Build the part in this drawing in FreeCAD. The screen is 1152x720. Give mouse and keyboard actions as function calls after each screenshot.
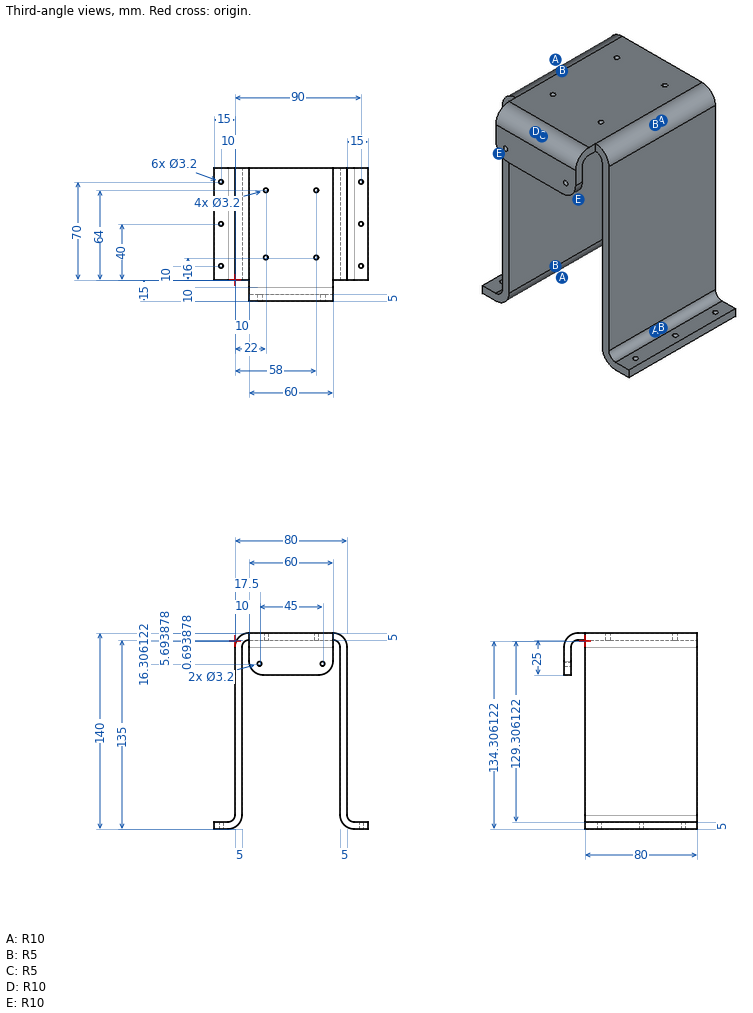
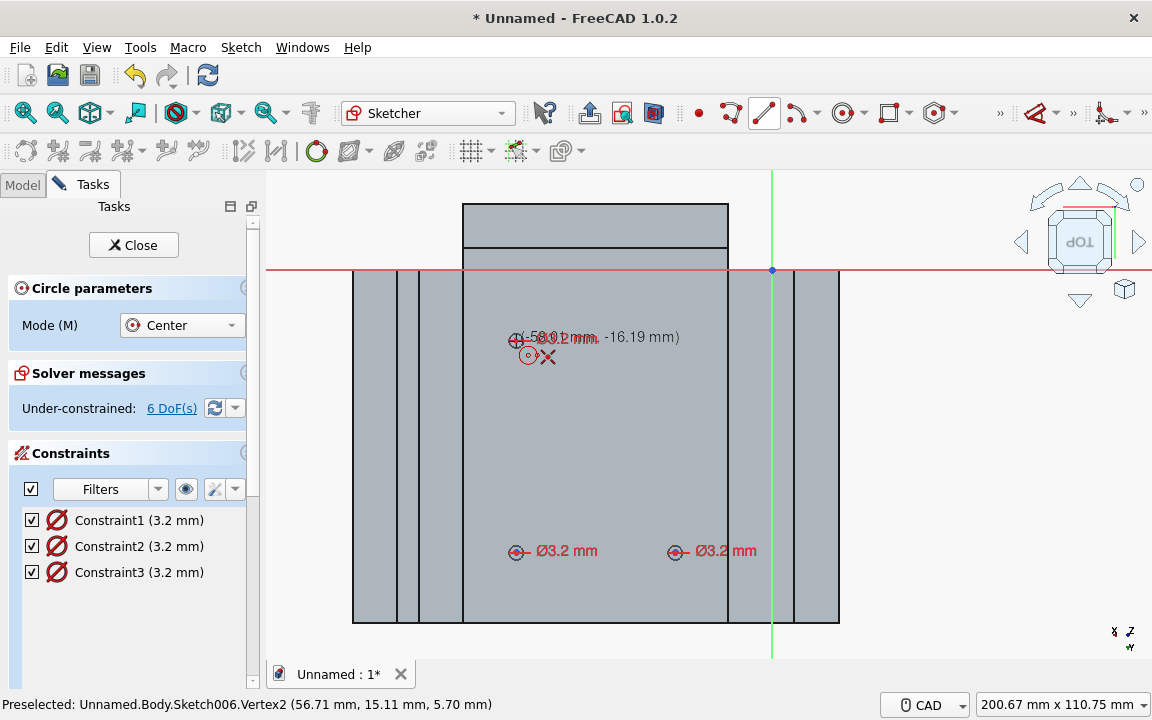
scroll(675, 341, up, 6)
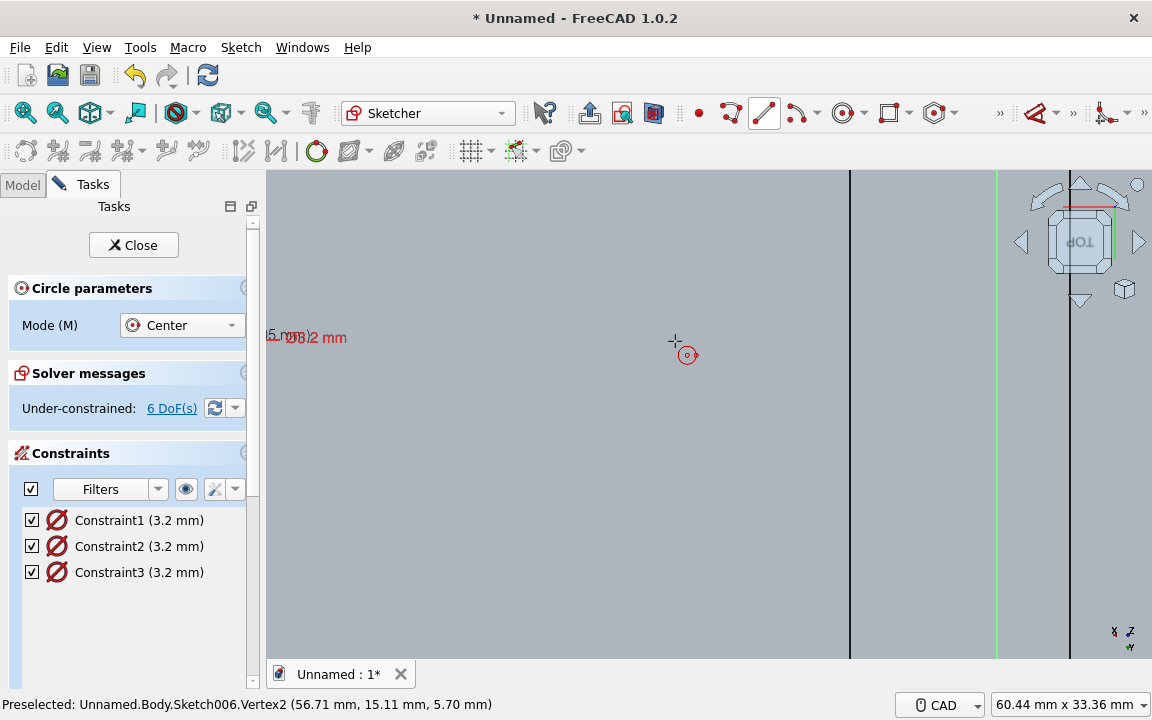
click(675, 339)
move(691, 323)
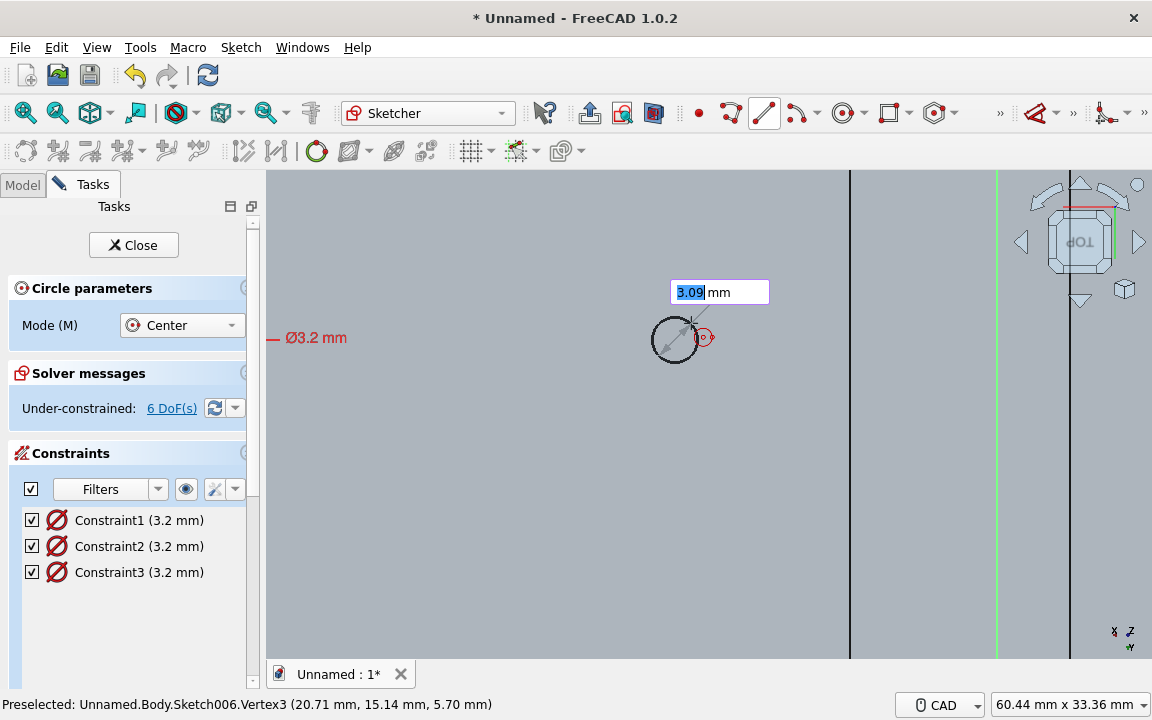
text(3.2)
key(Return)
key(Escape)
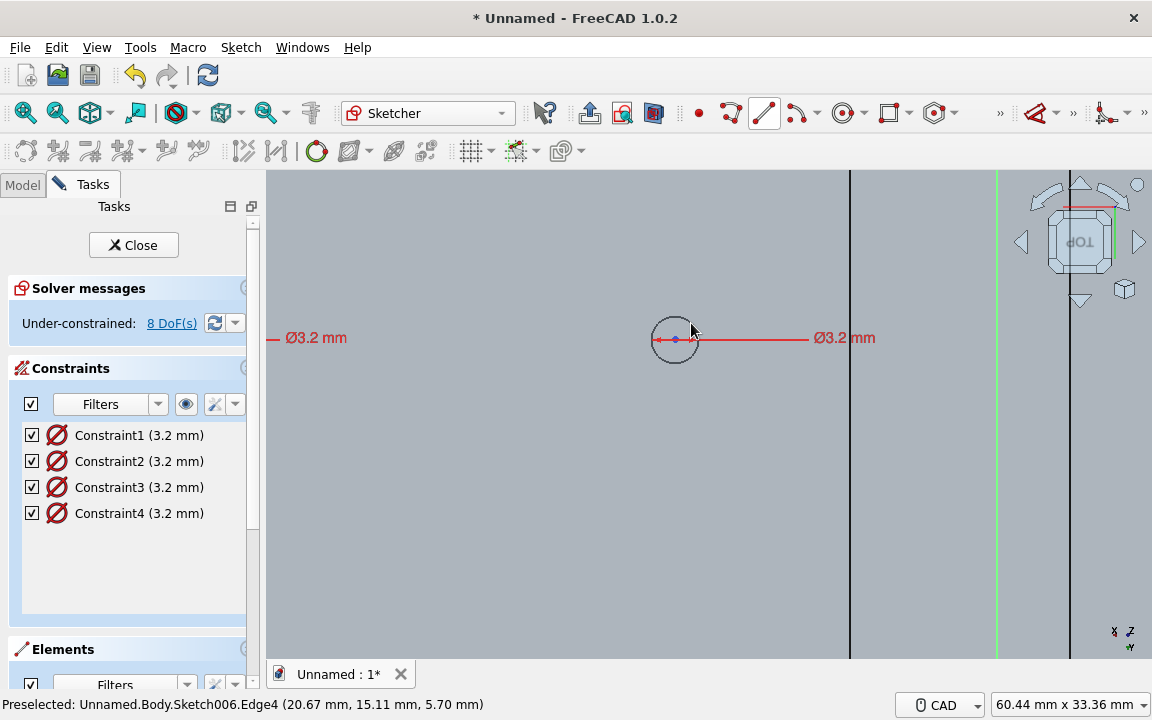
click(1036, 114)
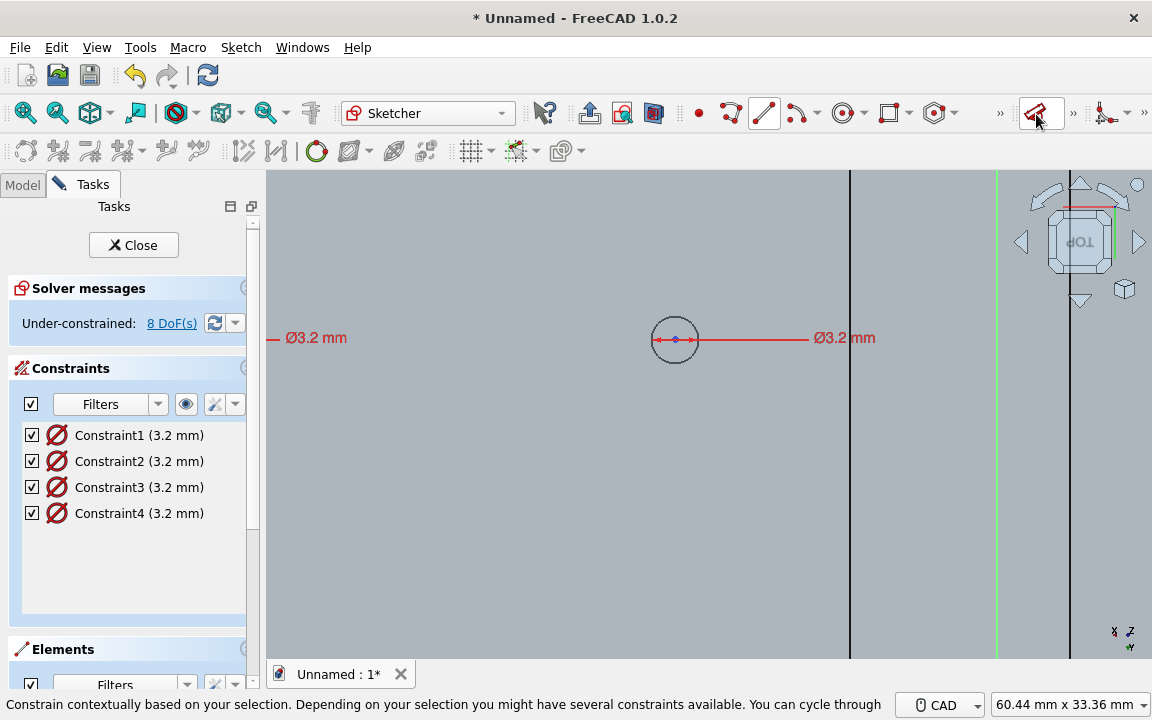
scroll(675, 341, down, 6)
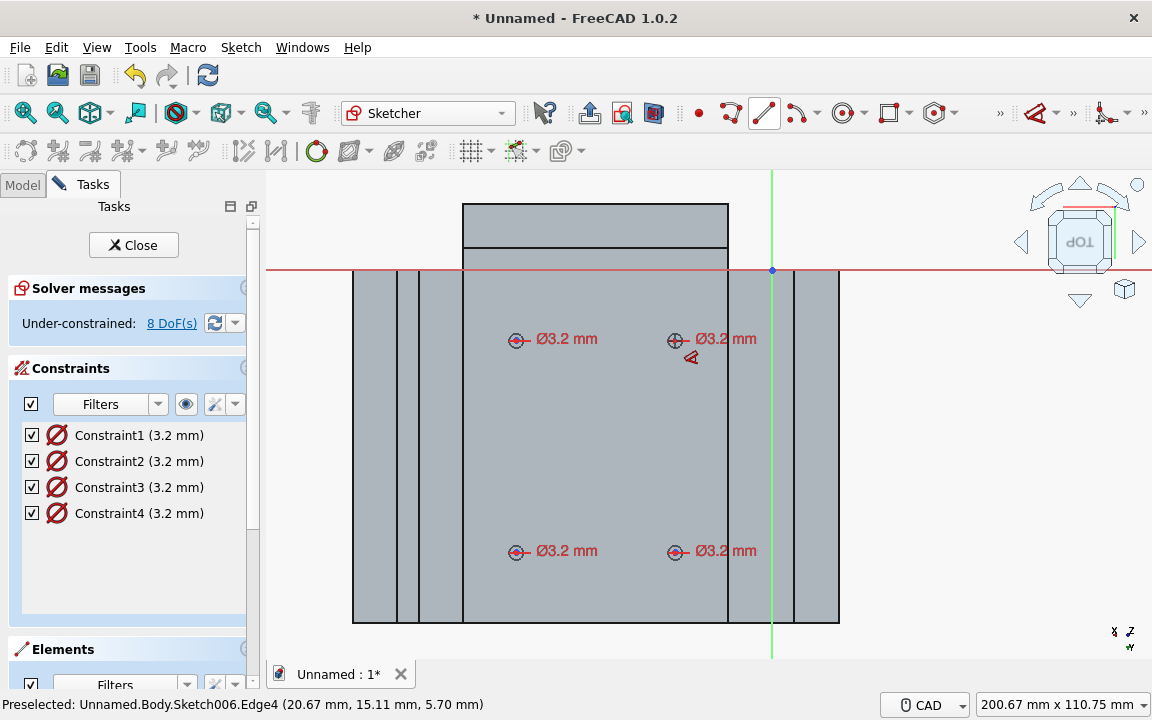
click(675, 553)
click(724, 236)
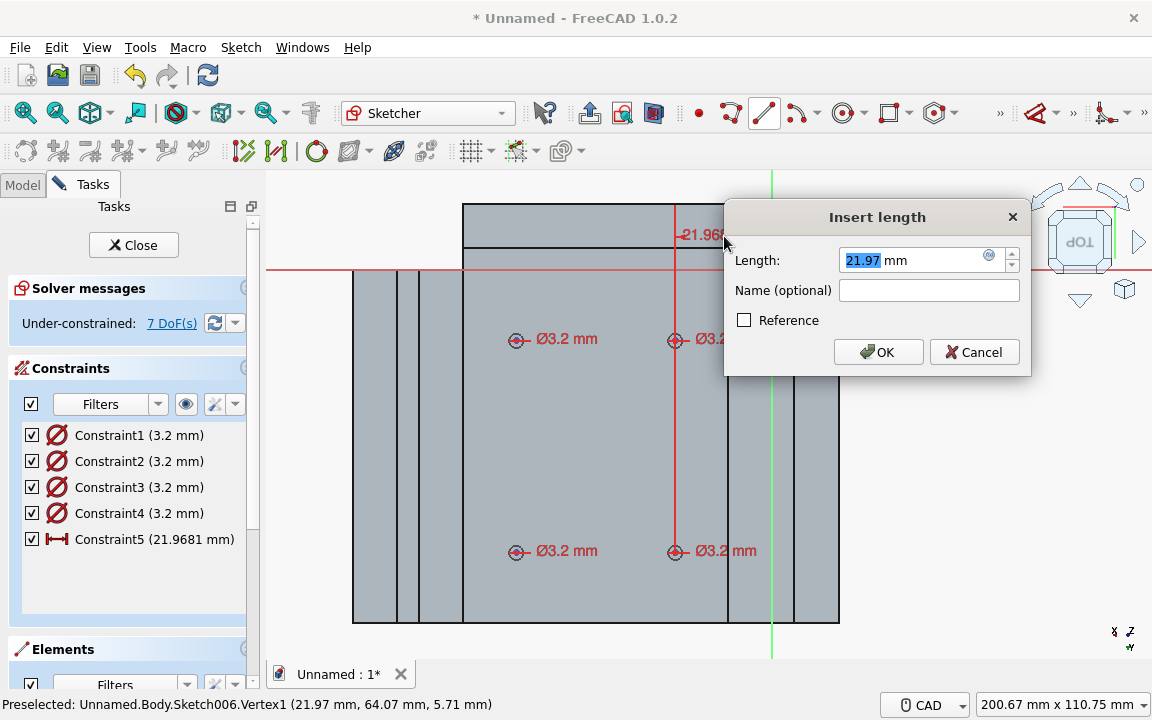
text(22)
key(Return)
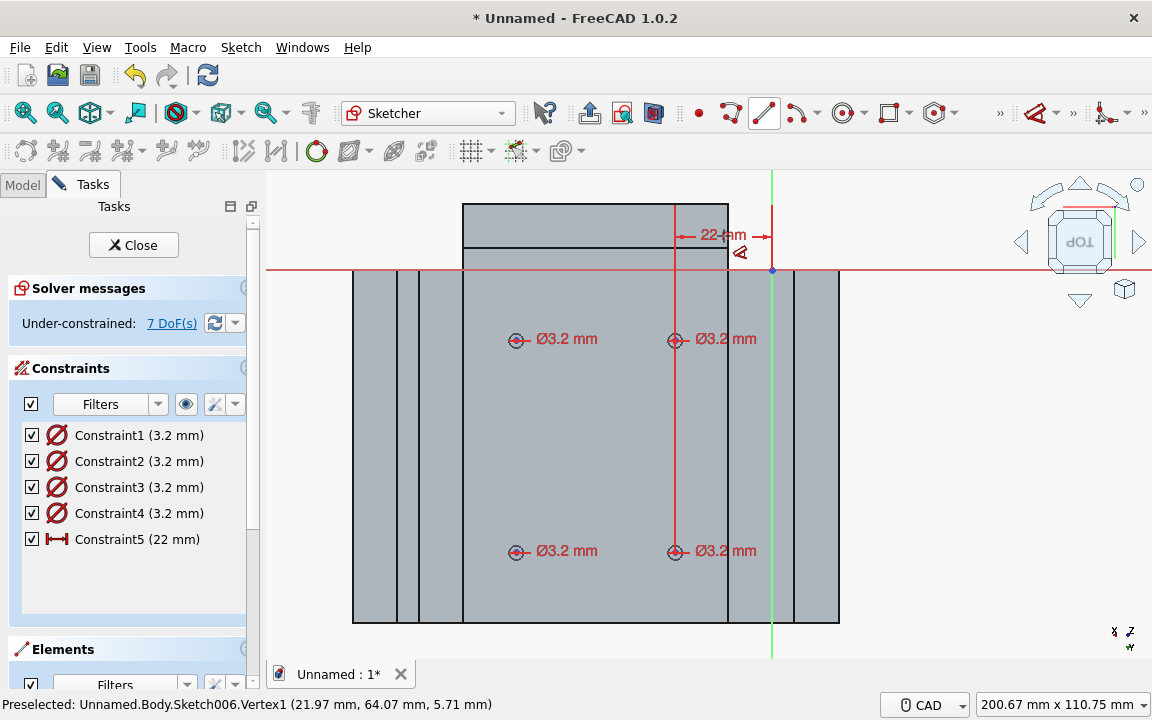
click(675, 553)
click(806, 412)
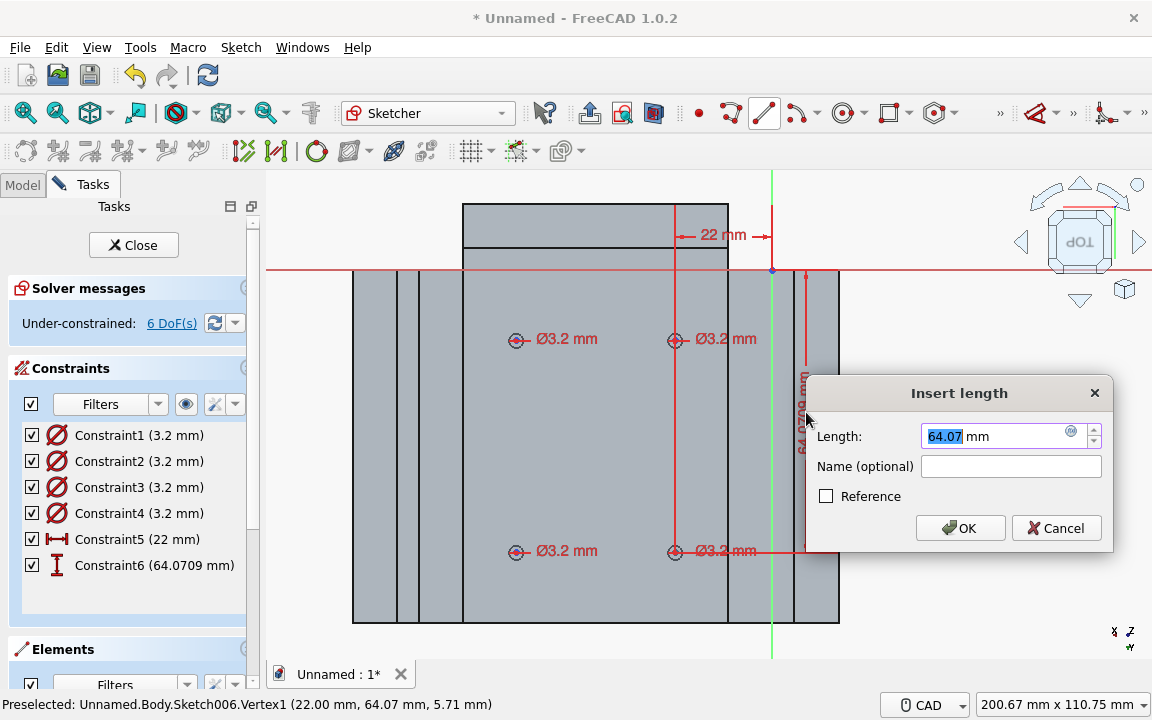
text(64)
key(Return)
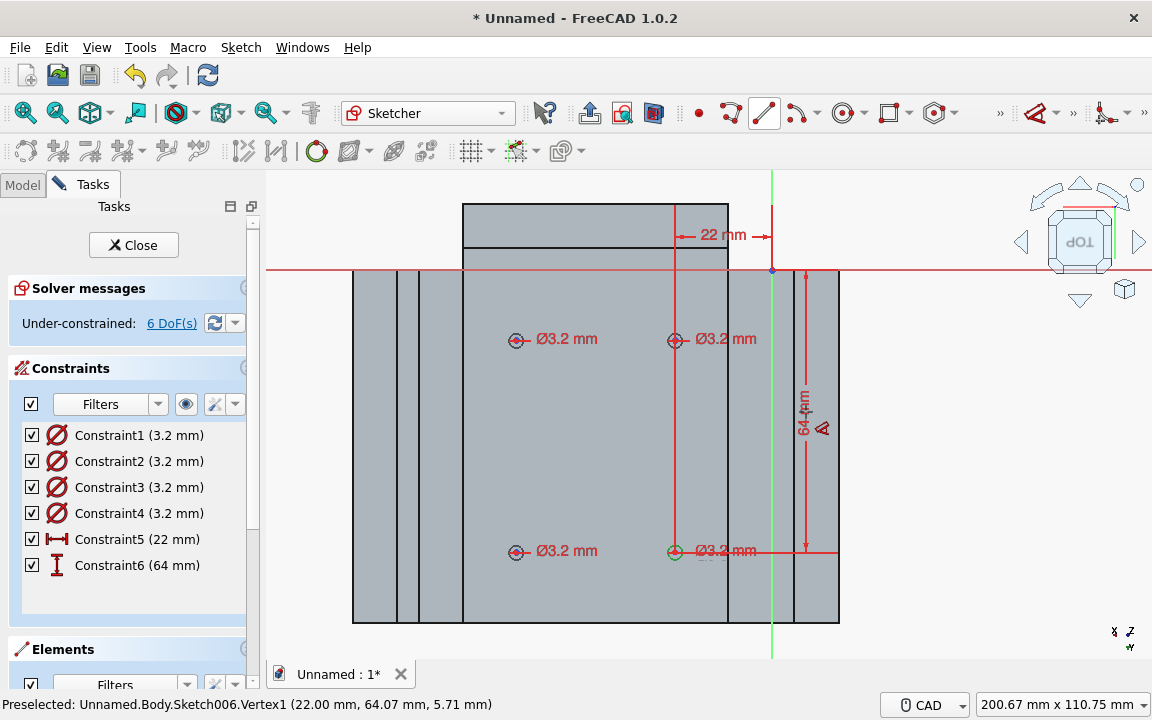
click(516, 553)
click(644, 236)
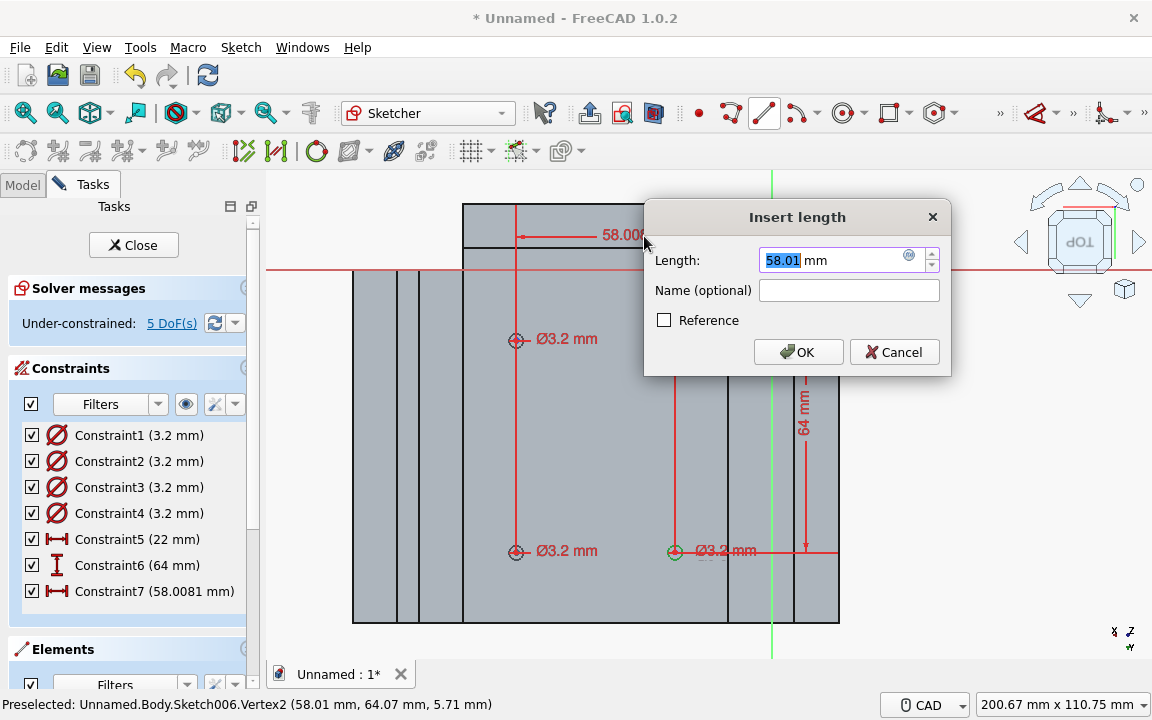
text(58)
key(Return)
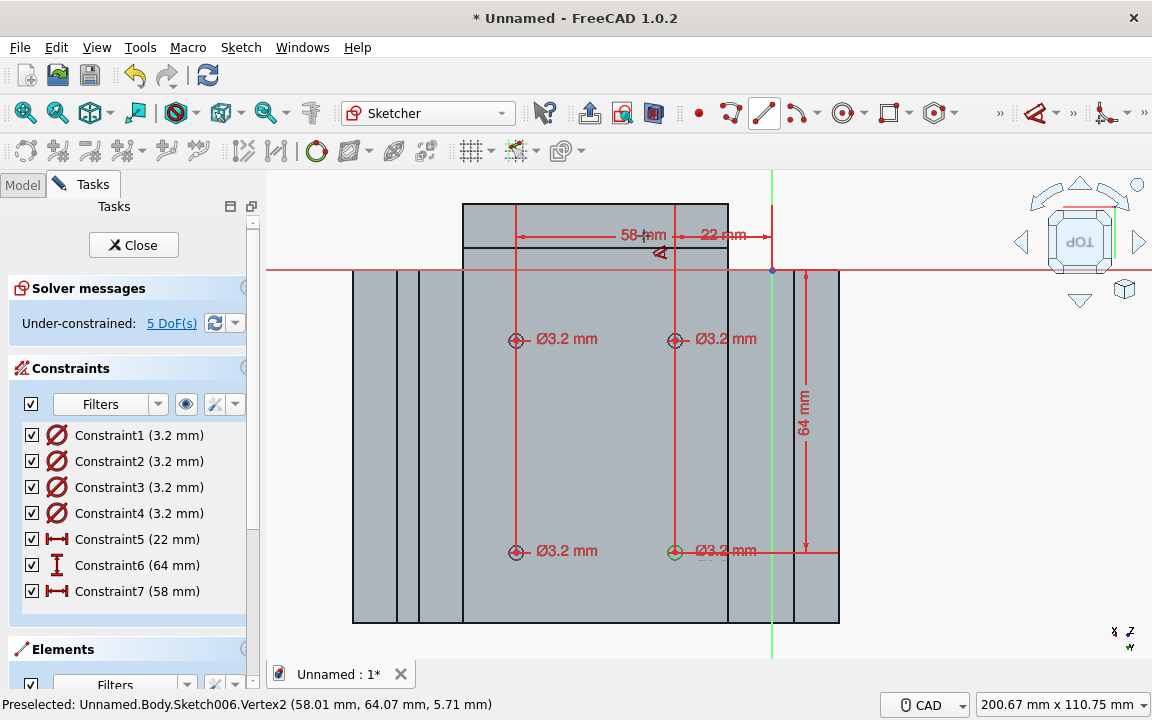
click(516, 553)
click(806, 346)